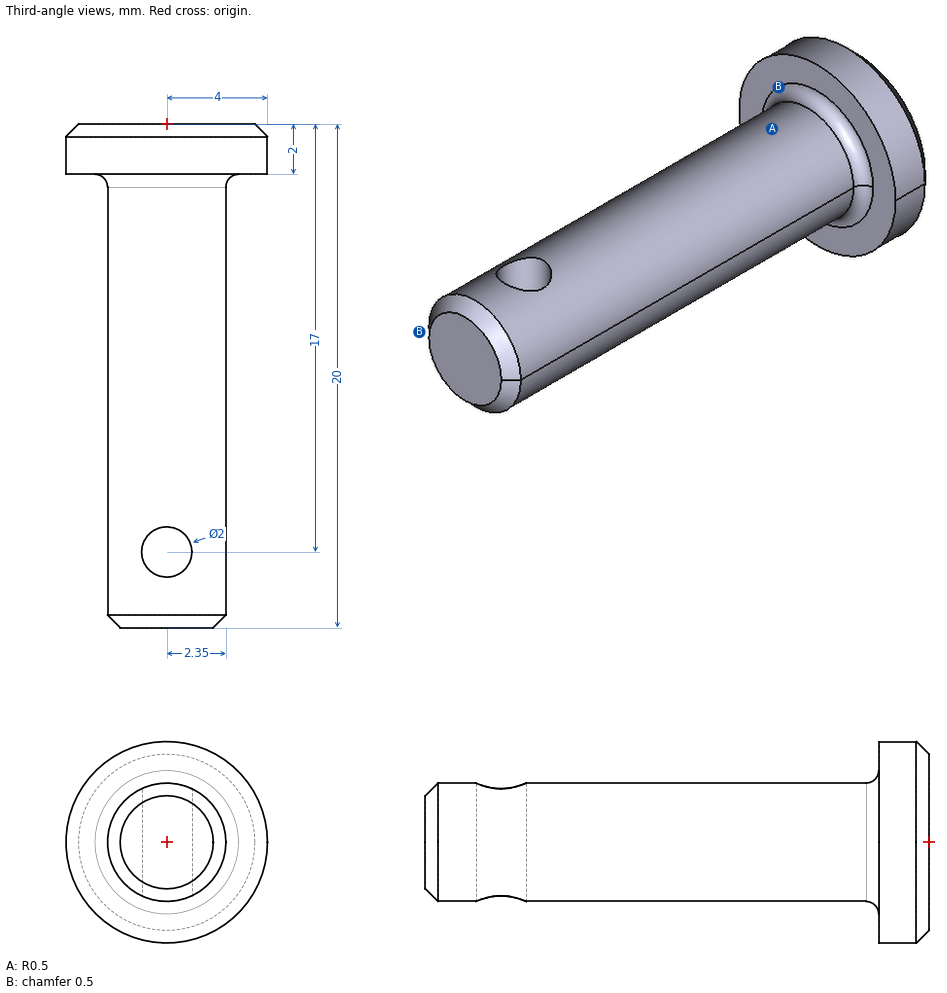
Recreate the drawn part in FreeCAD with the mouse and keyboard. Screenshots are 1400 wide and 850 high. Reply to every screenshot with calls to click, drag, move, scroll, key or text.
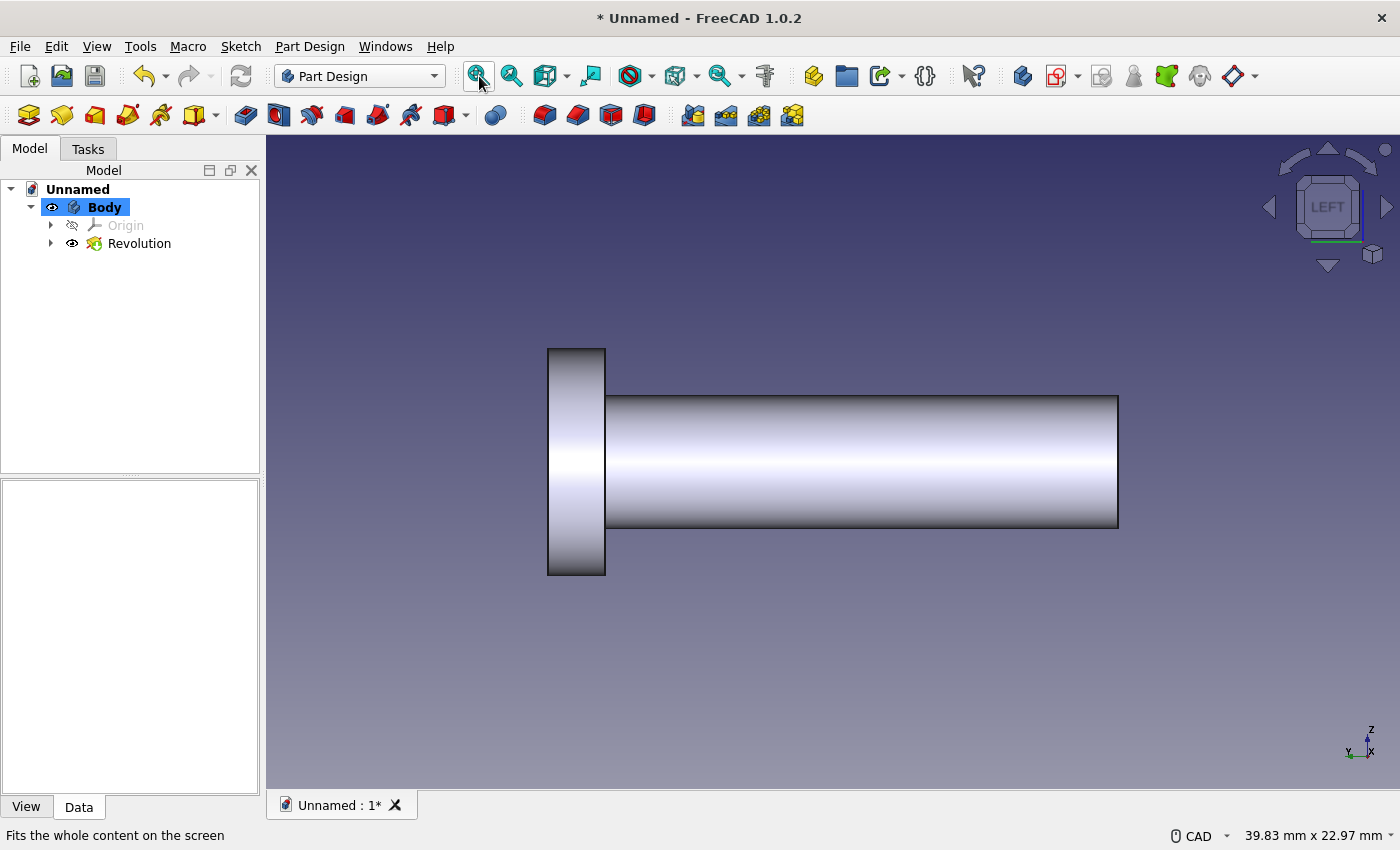
key(v)
key(3)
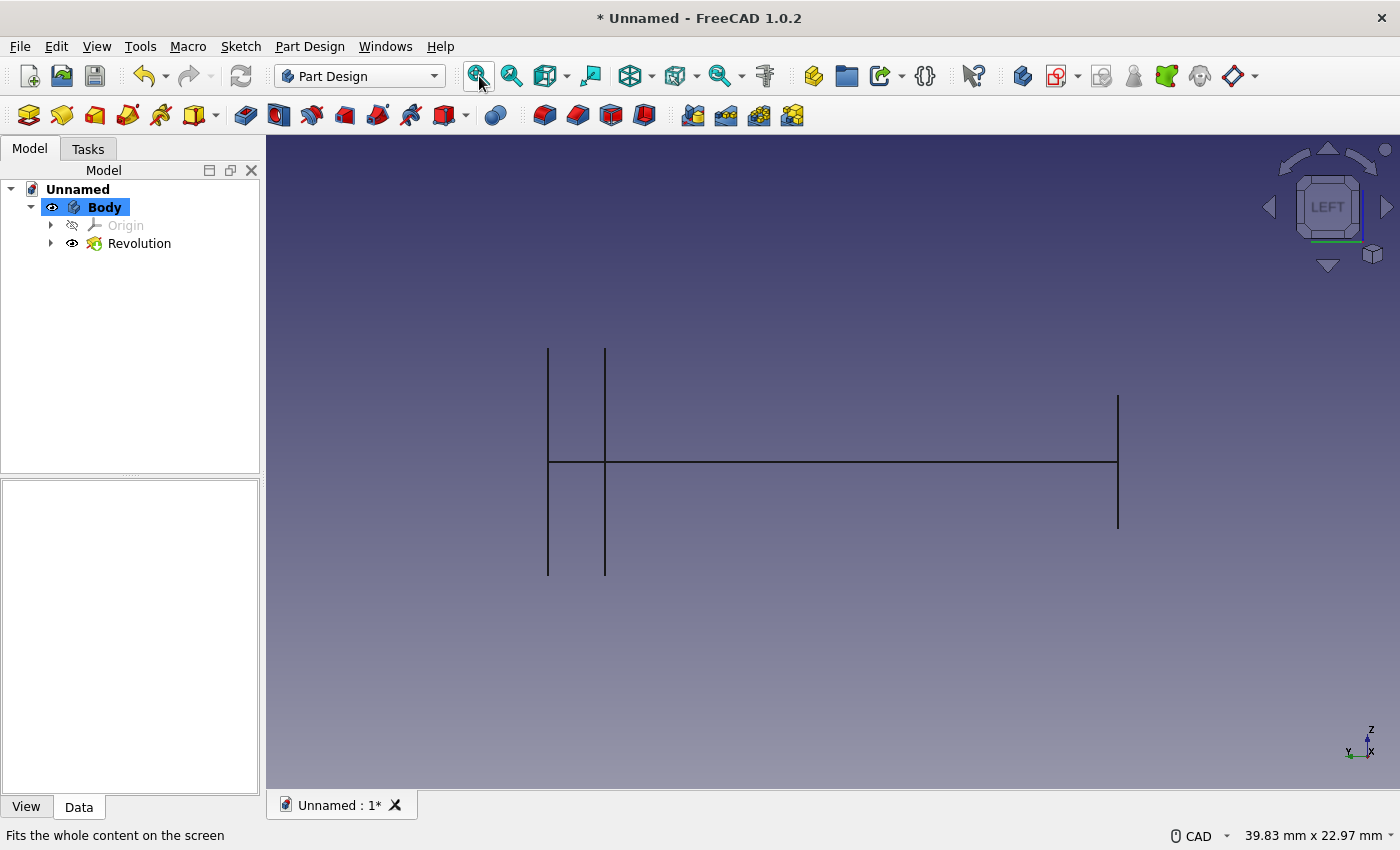
key(0)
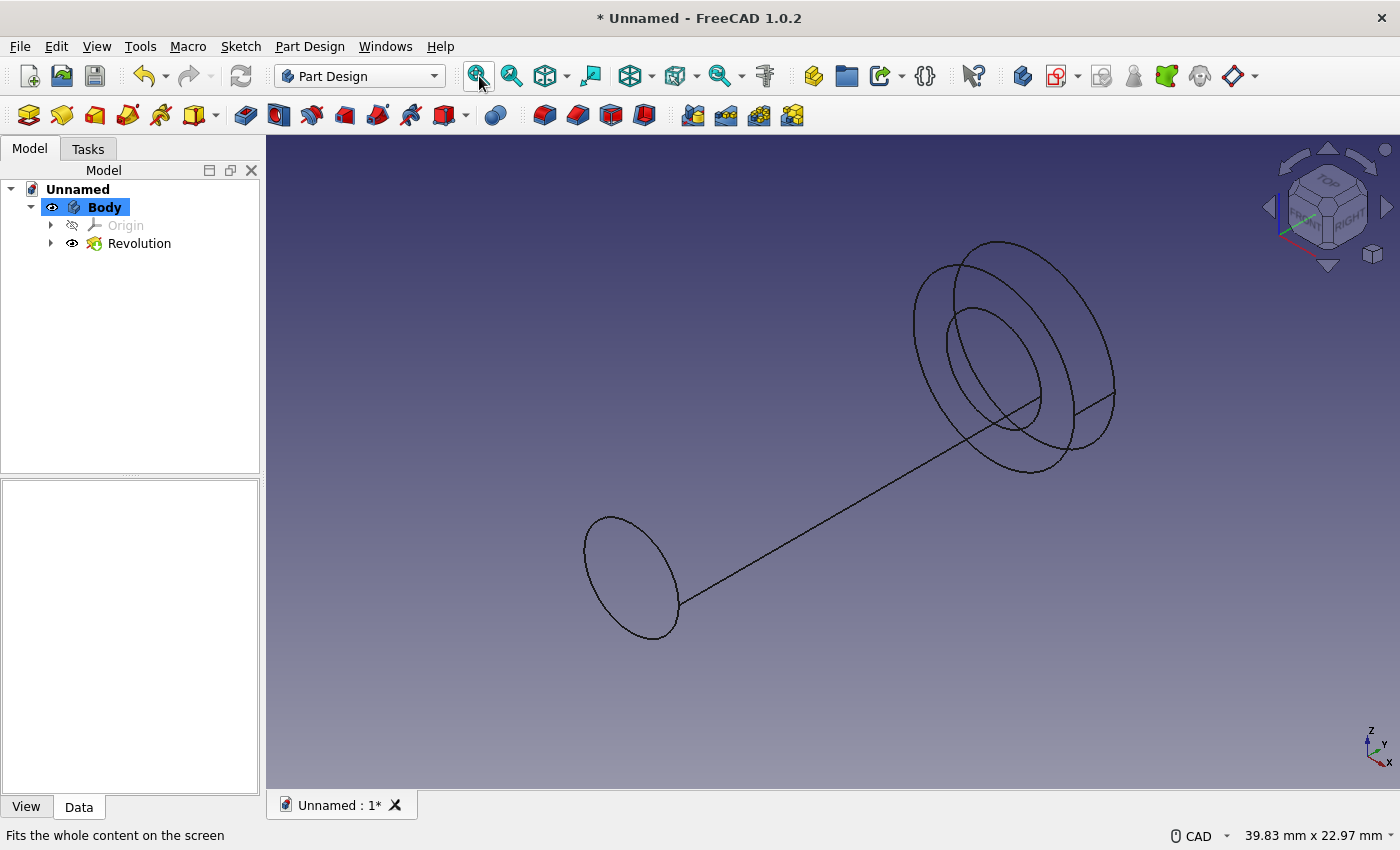
click(947, 341)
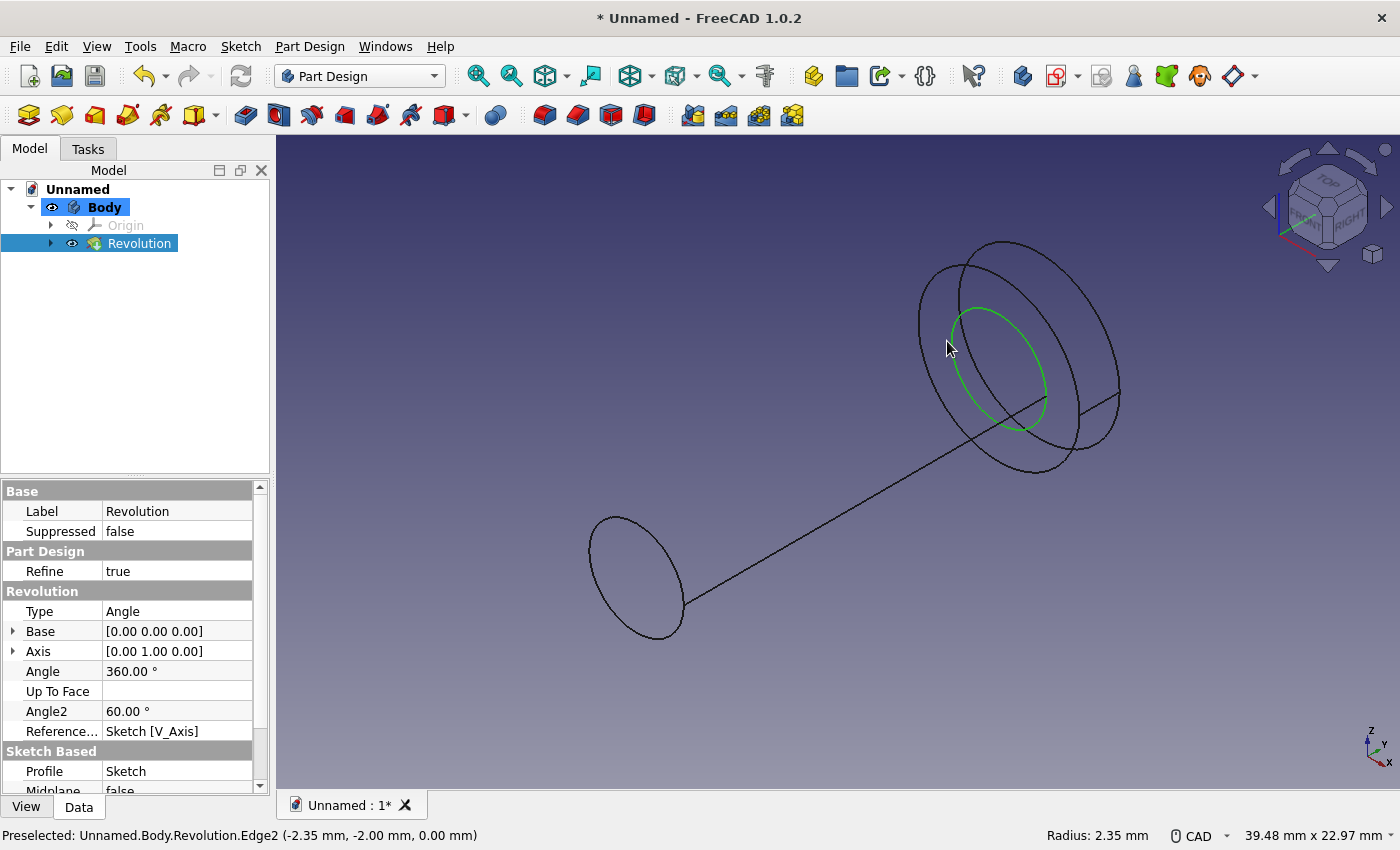
key(v)
key(1)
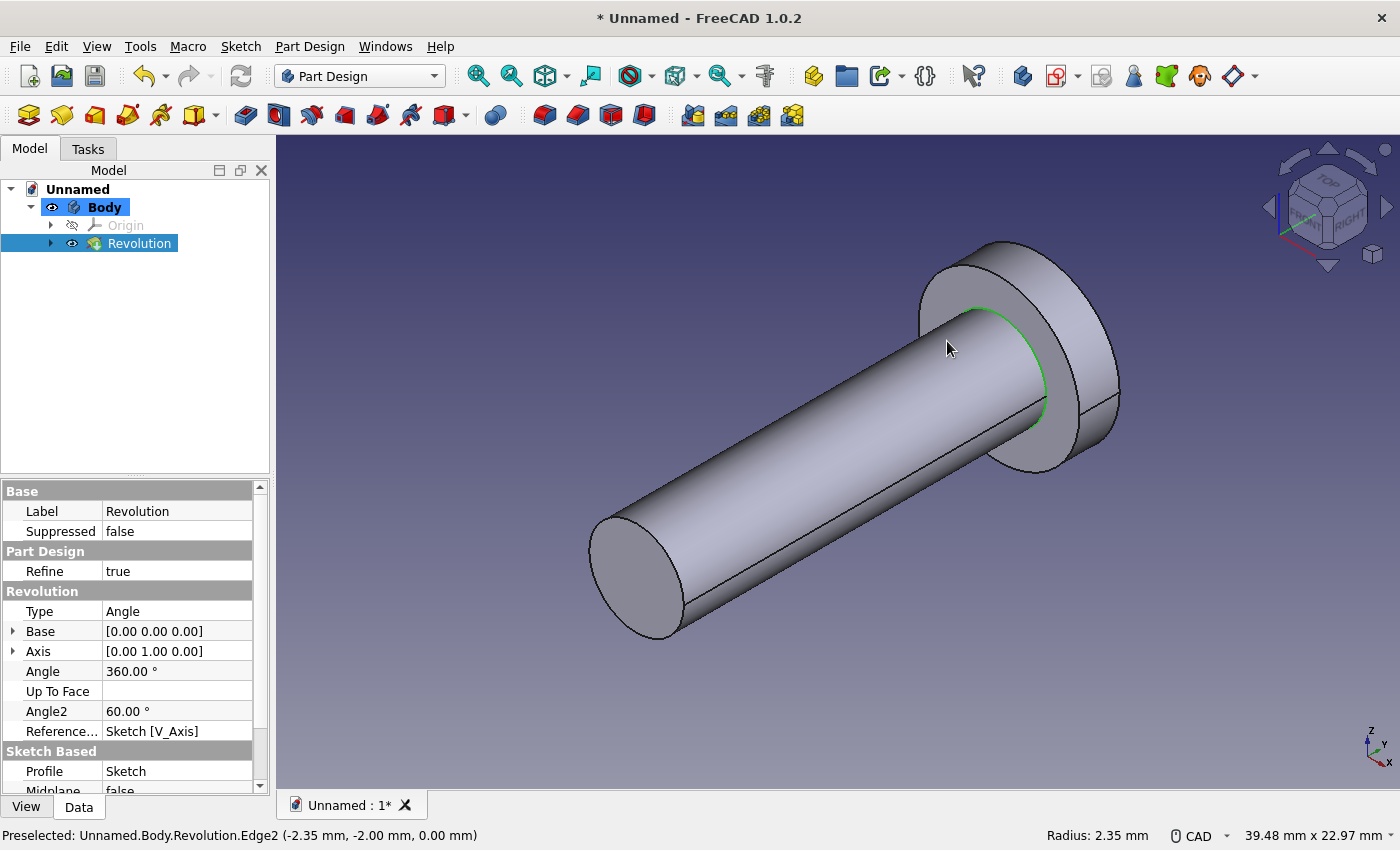
click(545, 116)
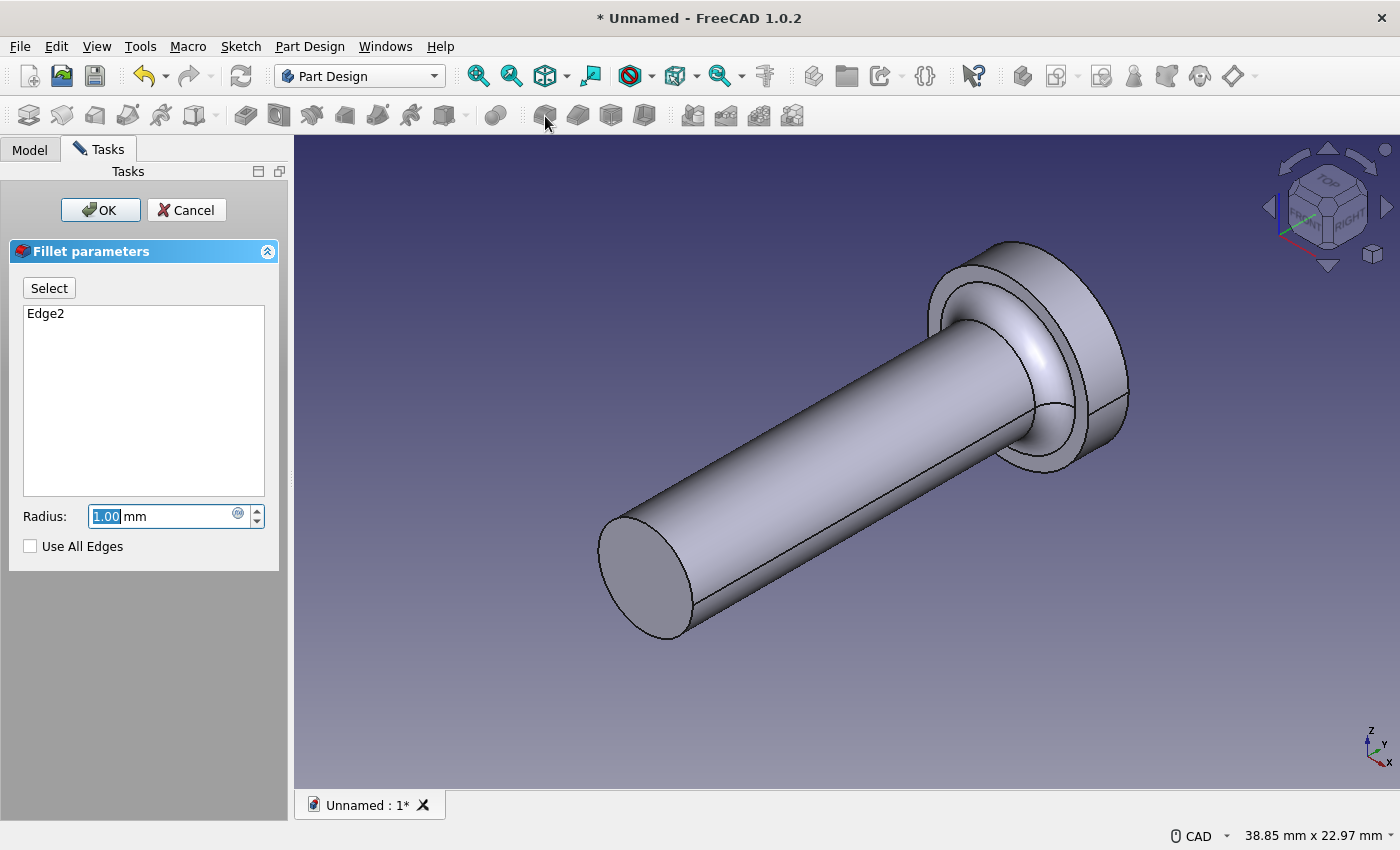
text(0.5)
key(Tab)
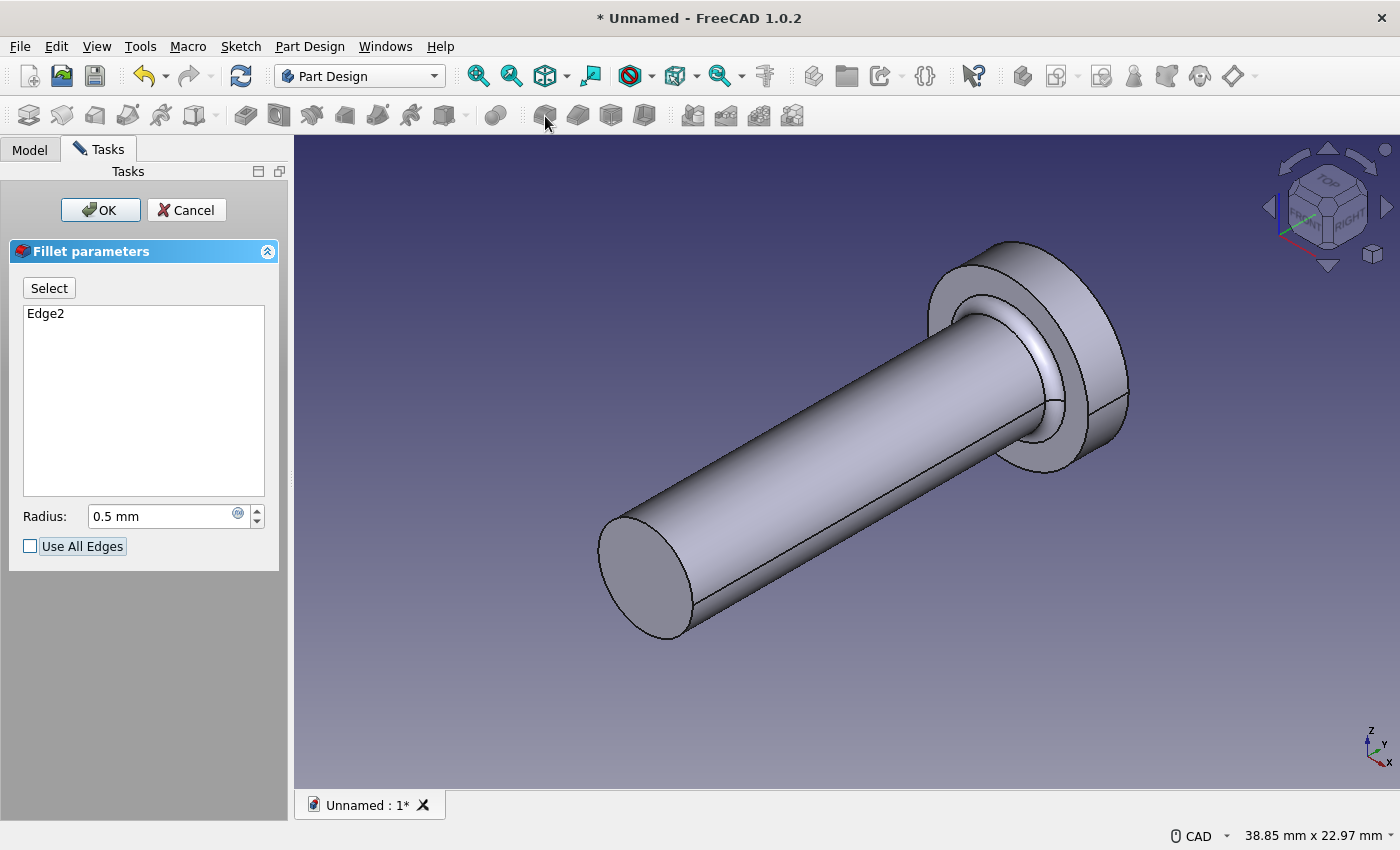
click(101, 210)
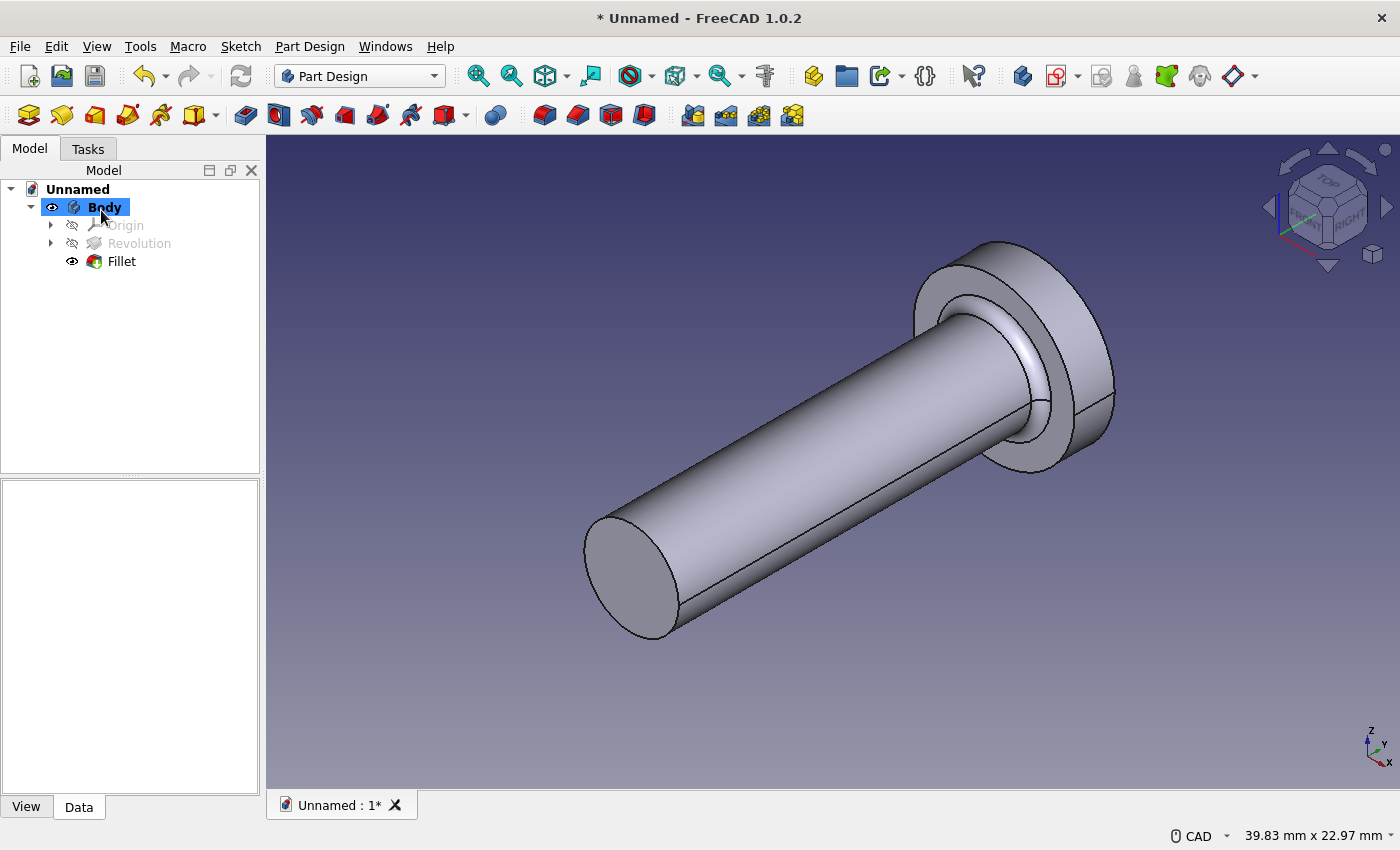
click(617, 517)